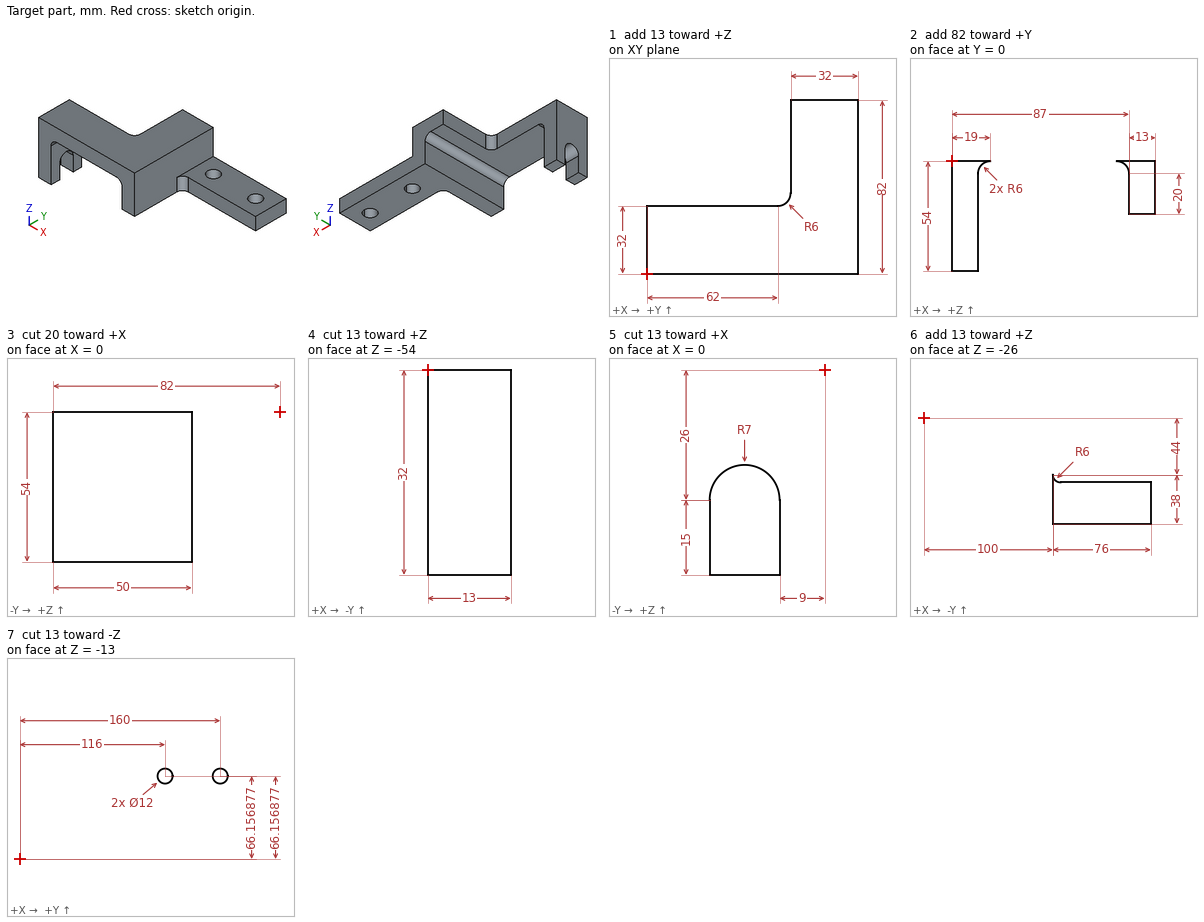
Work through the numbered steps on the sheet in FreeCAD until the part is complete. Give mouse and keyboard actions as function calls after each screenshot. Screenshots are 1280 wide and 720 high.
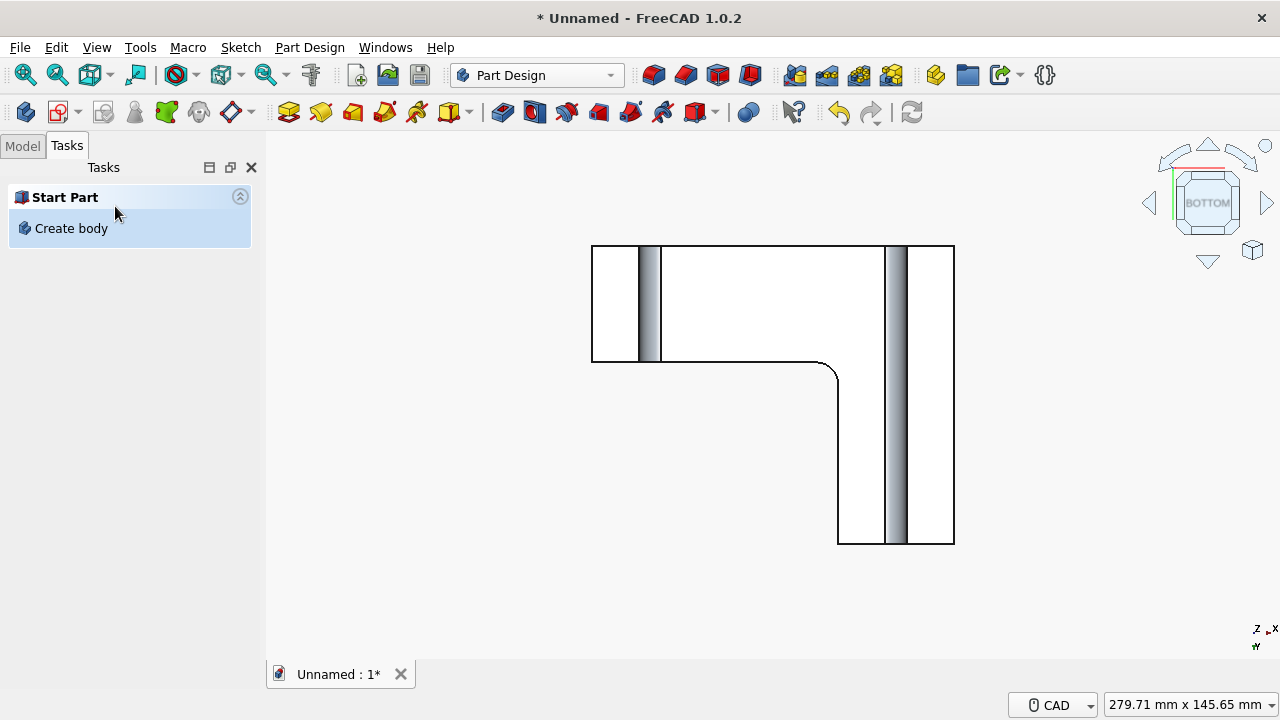
click(615, 337)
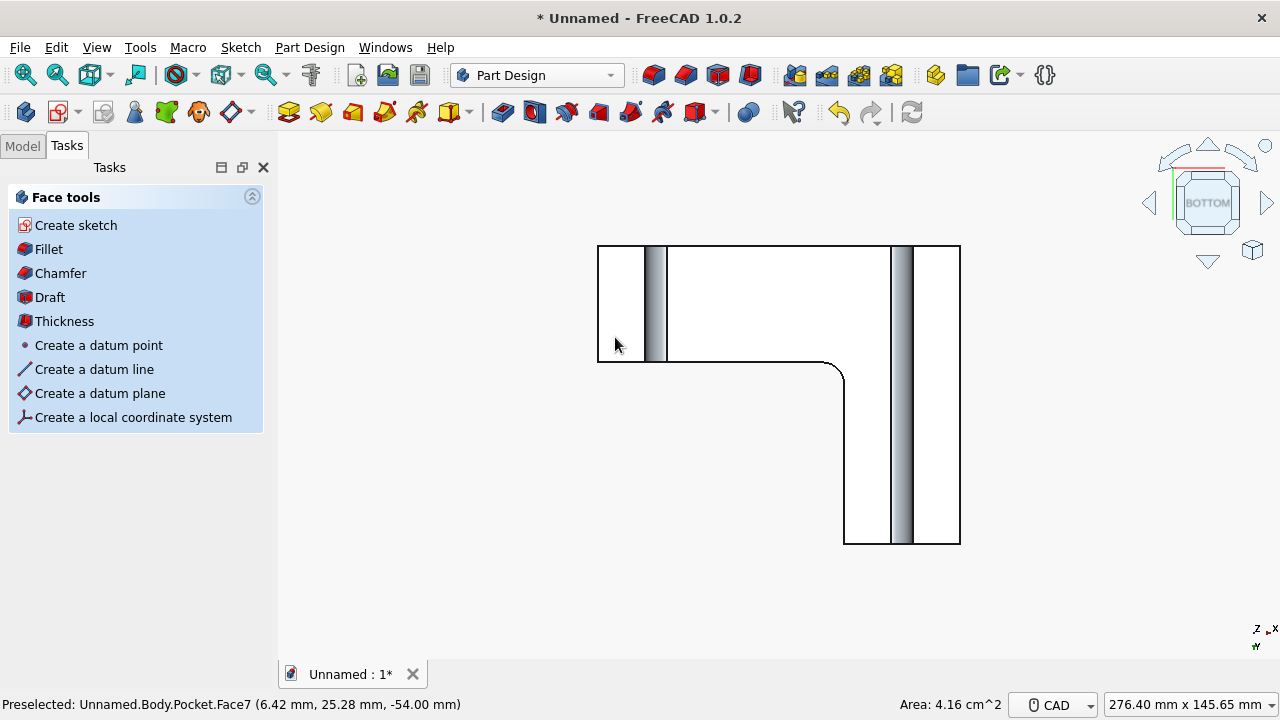
click(58, 112)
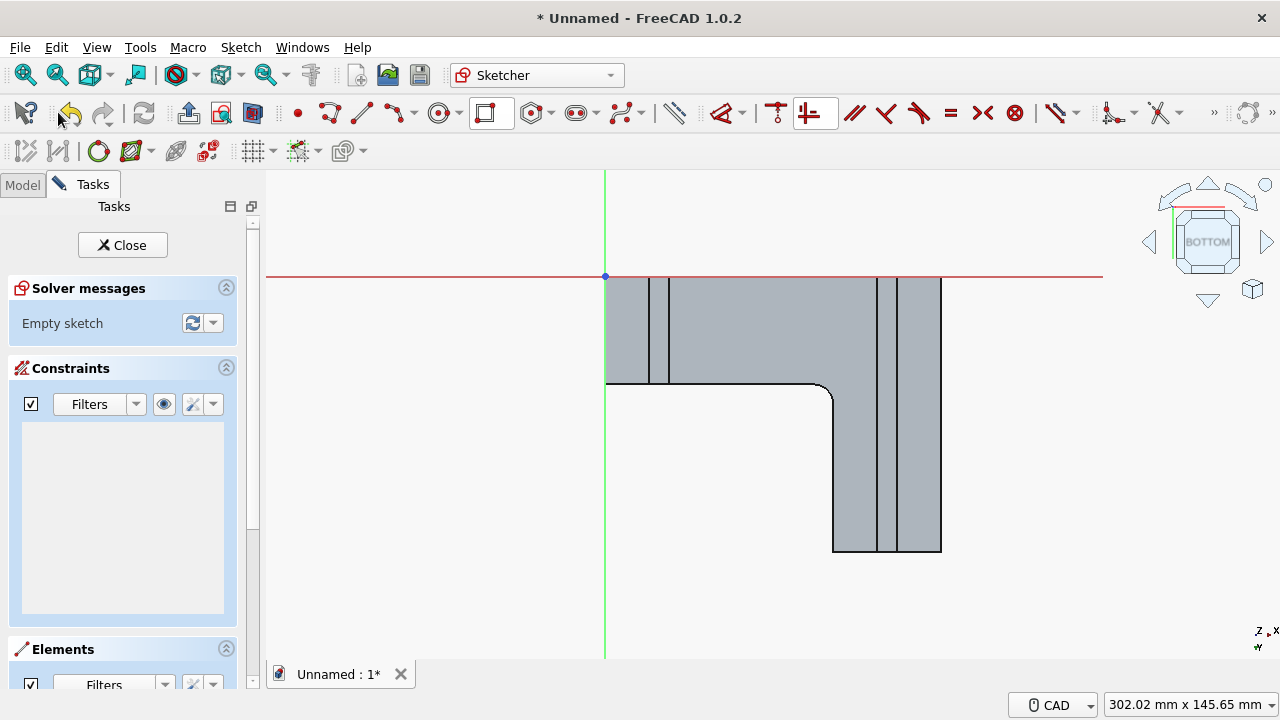
scroll(582, 282, up, 5)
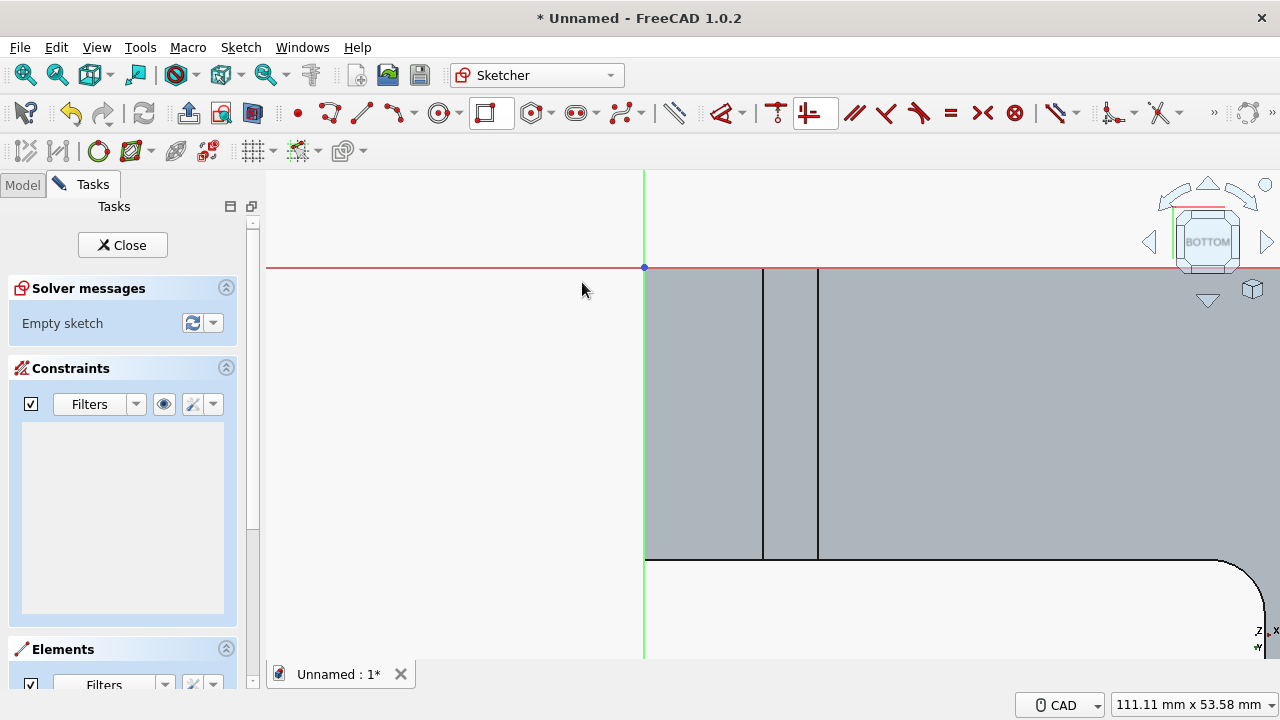
click(486, 114)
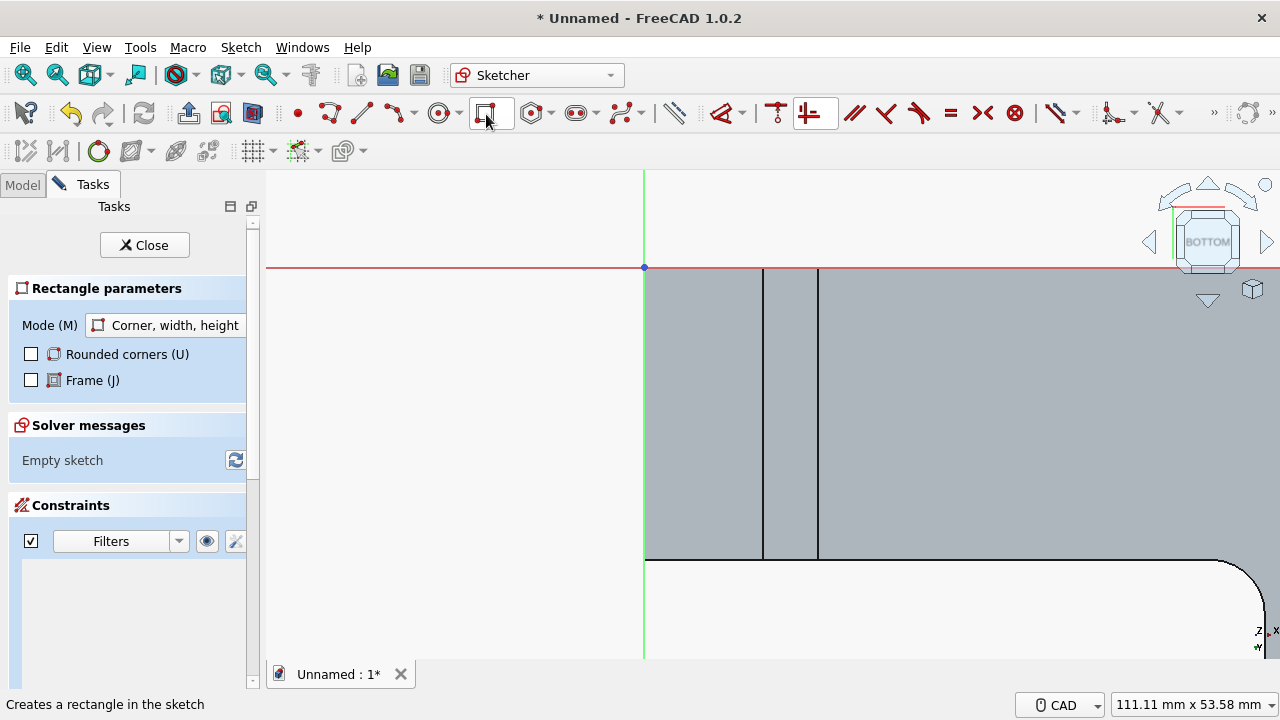
click(644, 268)
click(763, 560)
key(Escape)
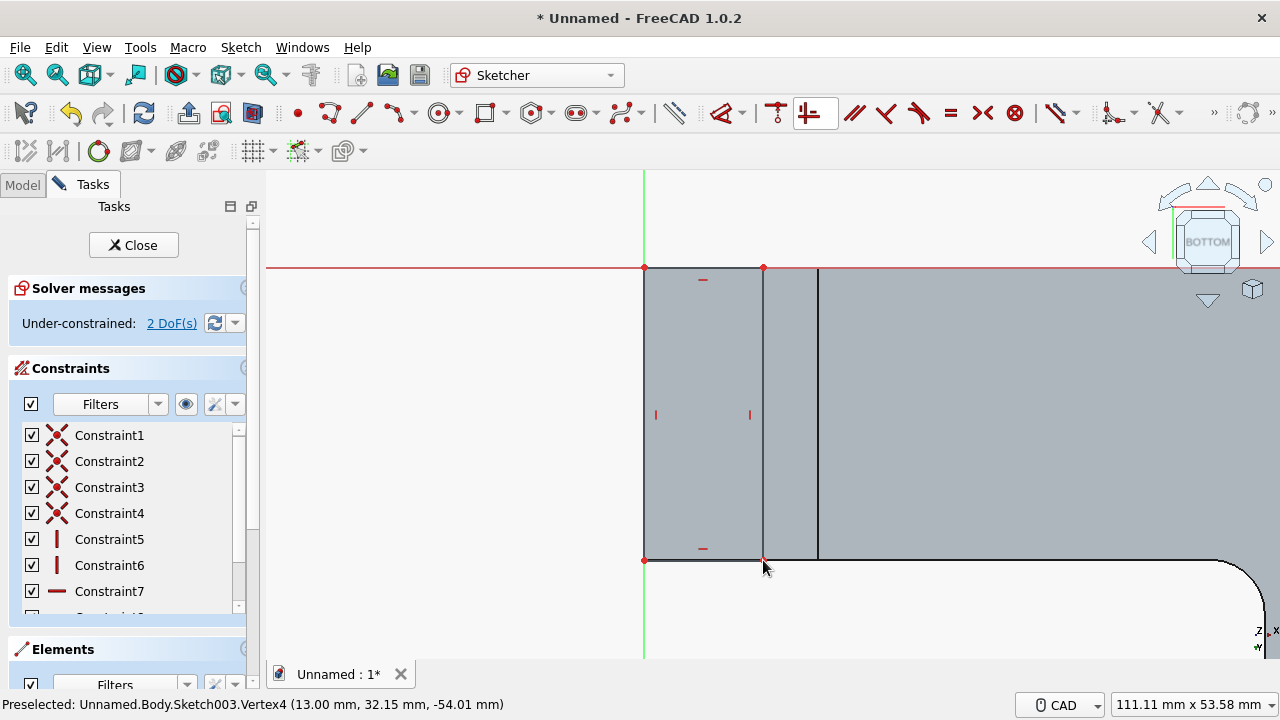
click(722, 114)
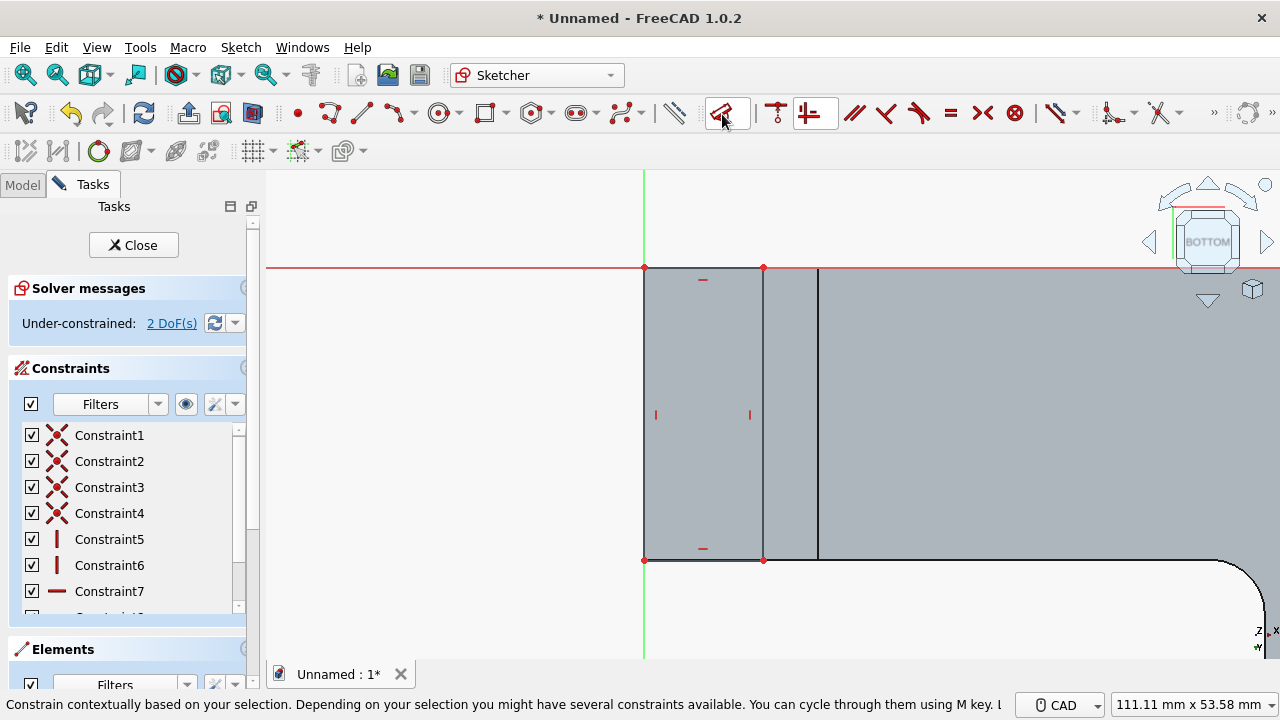
click(644, 356)
click(610, 414)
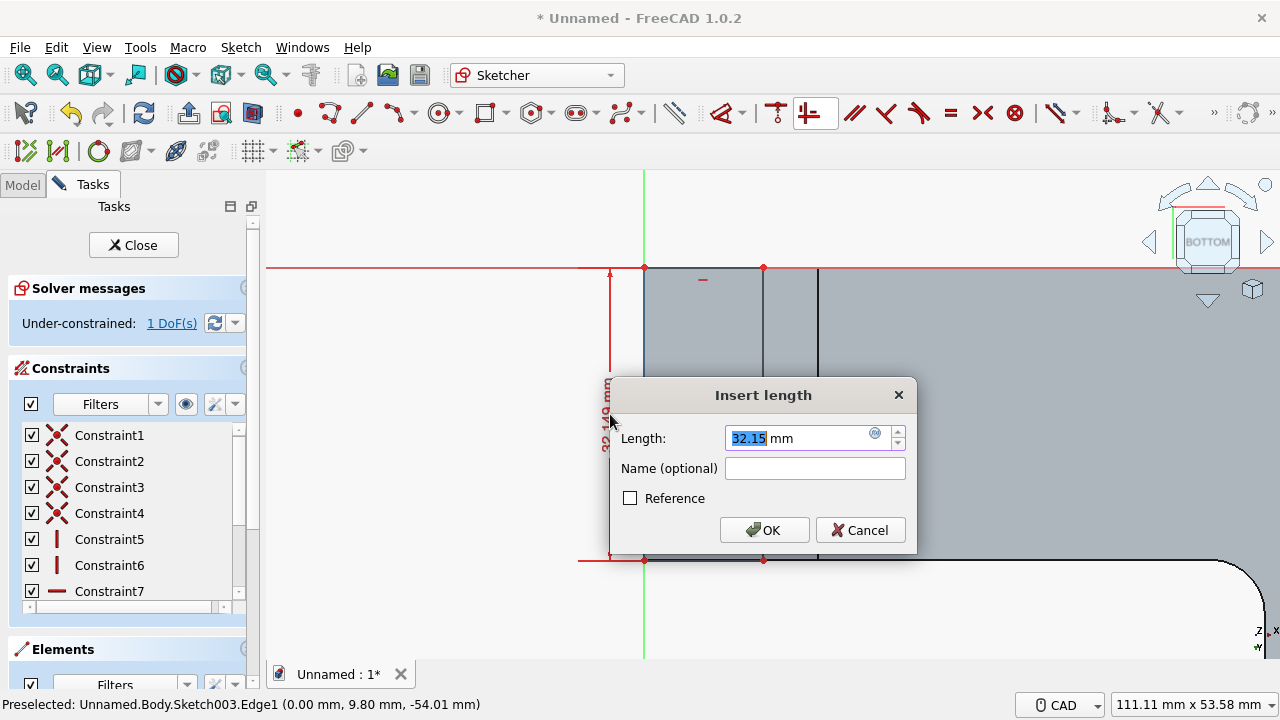
text(32)
key(Return)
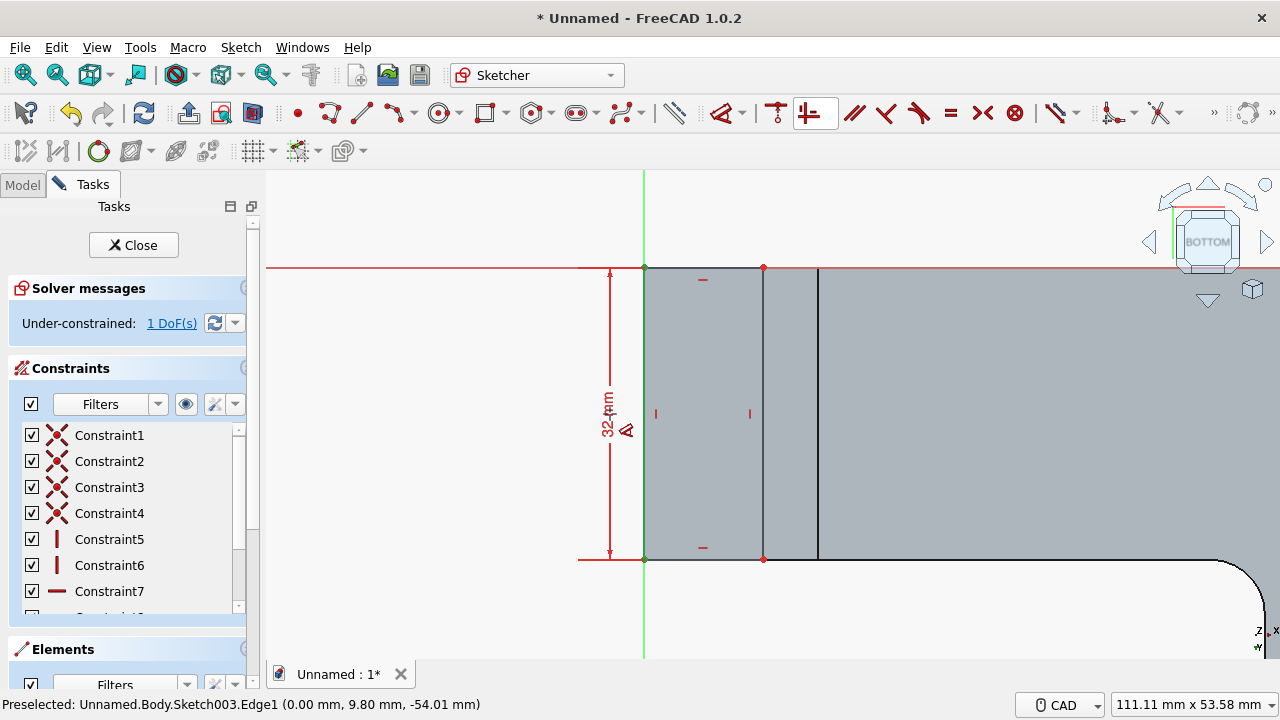
click(680, 560)
click(704, 594)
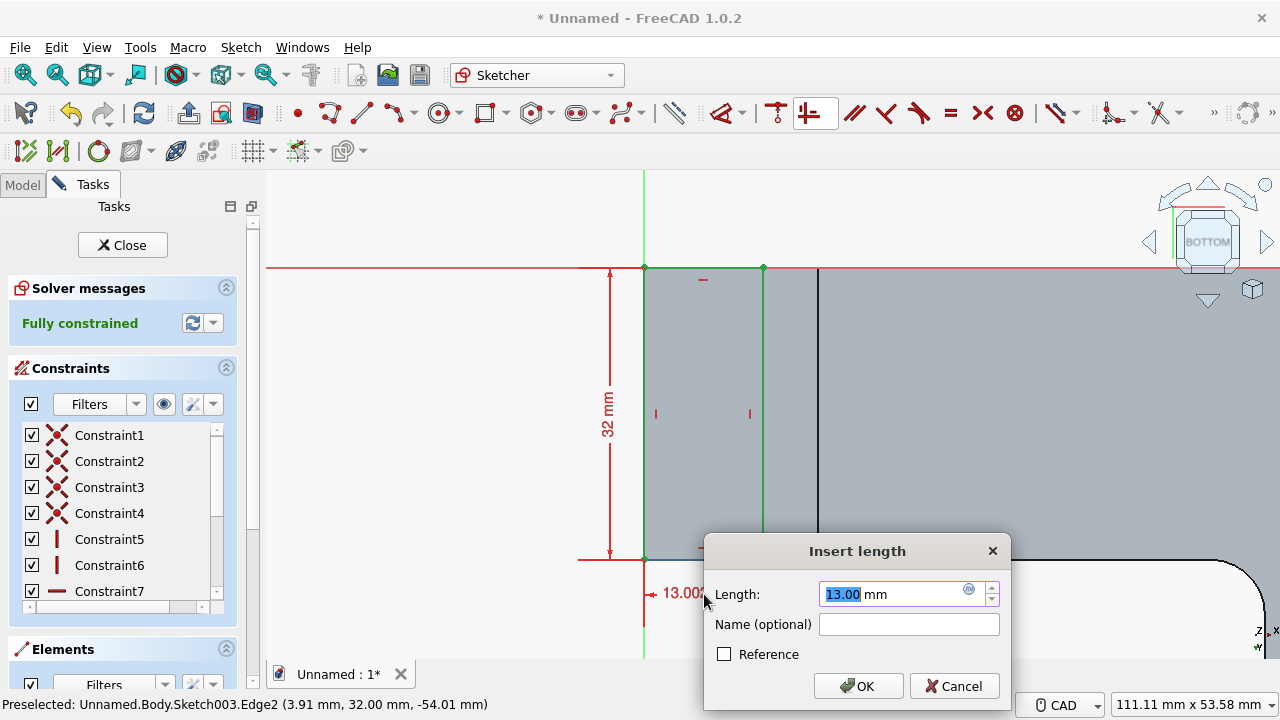
text(13)
key(Return)
key(Escape)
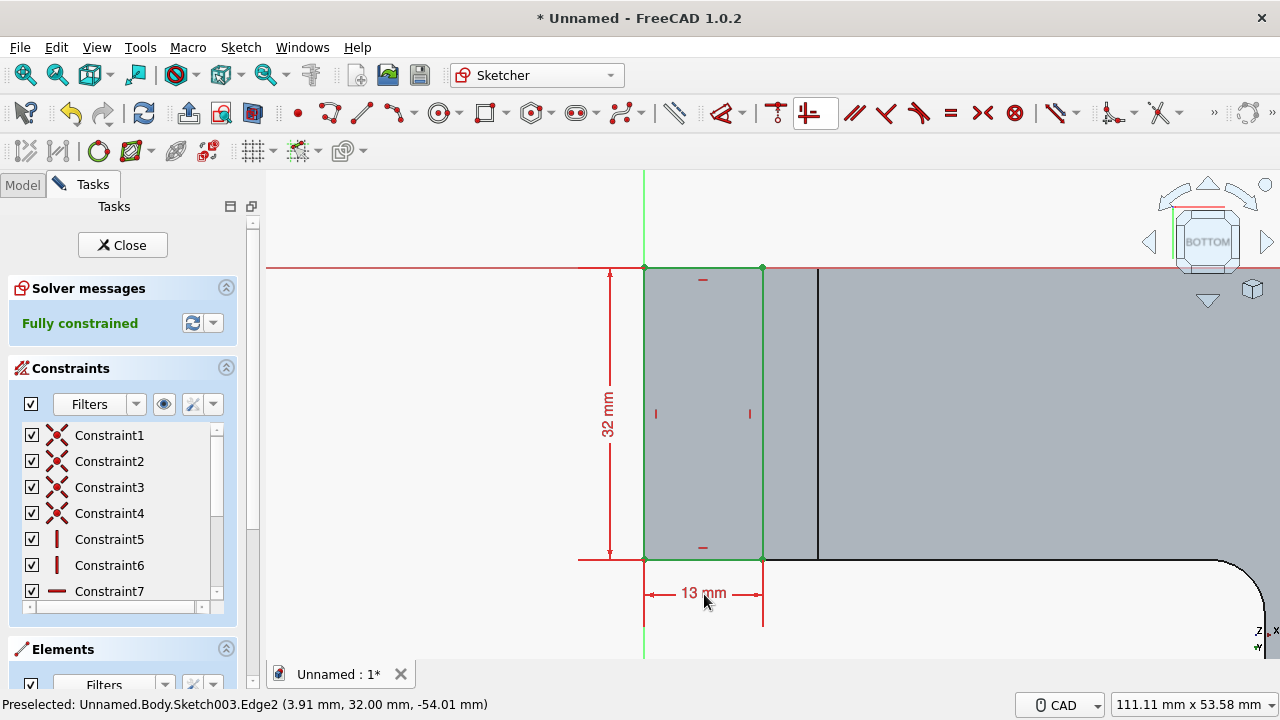
click(123, 245)